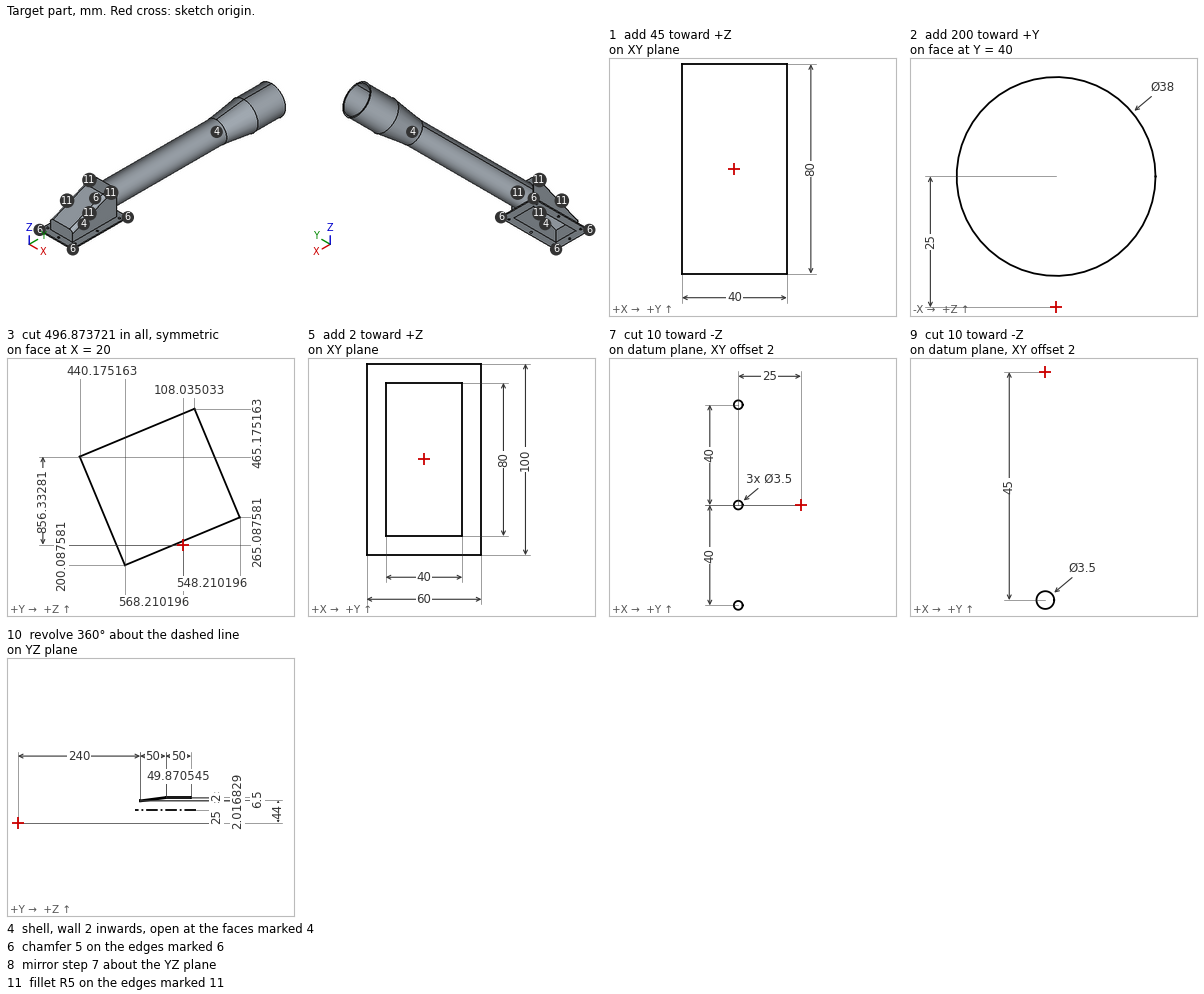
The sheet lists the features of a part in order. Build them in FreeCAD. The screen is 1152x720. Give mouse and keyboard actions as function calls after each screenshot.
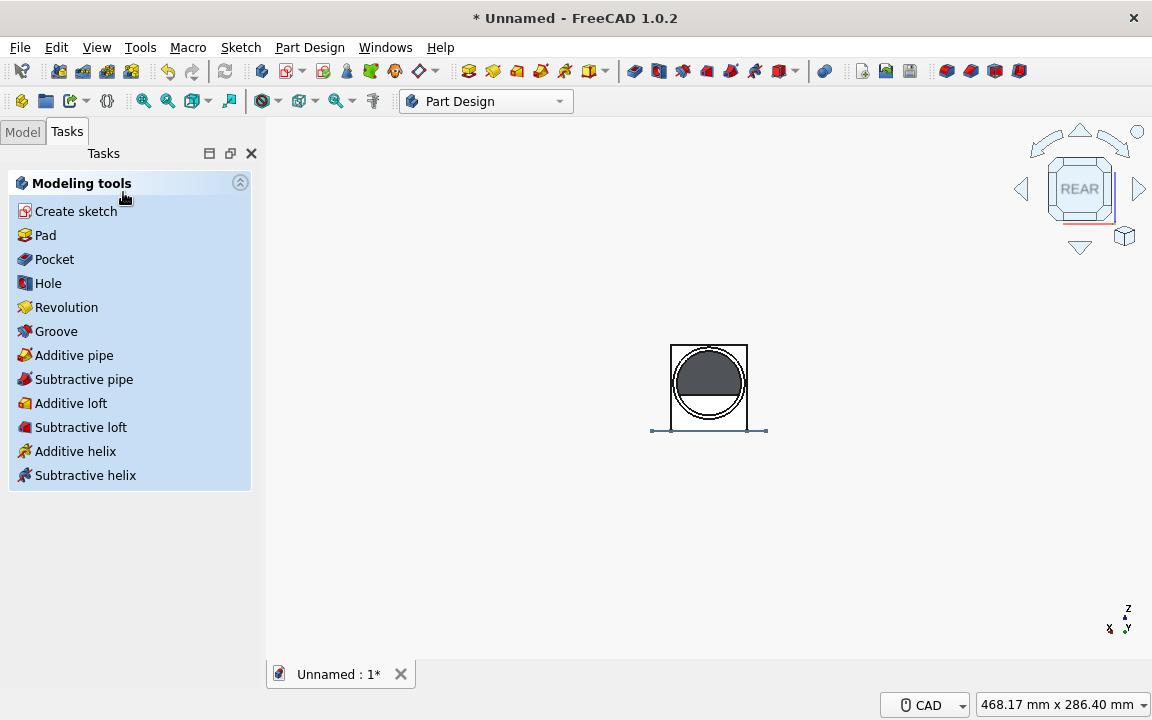
click(470, 72)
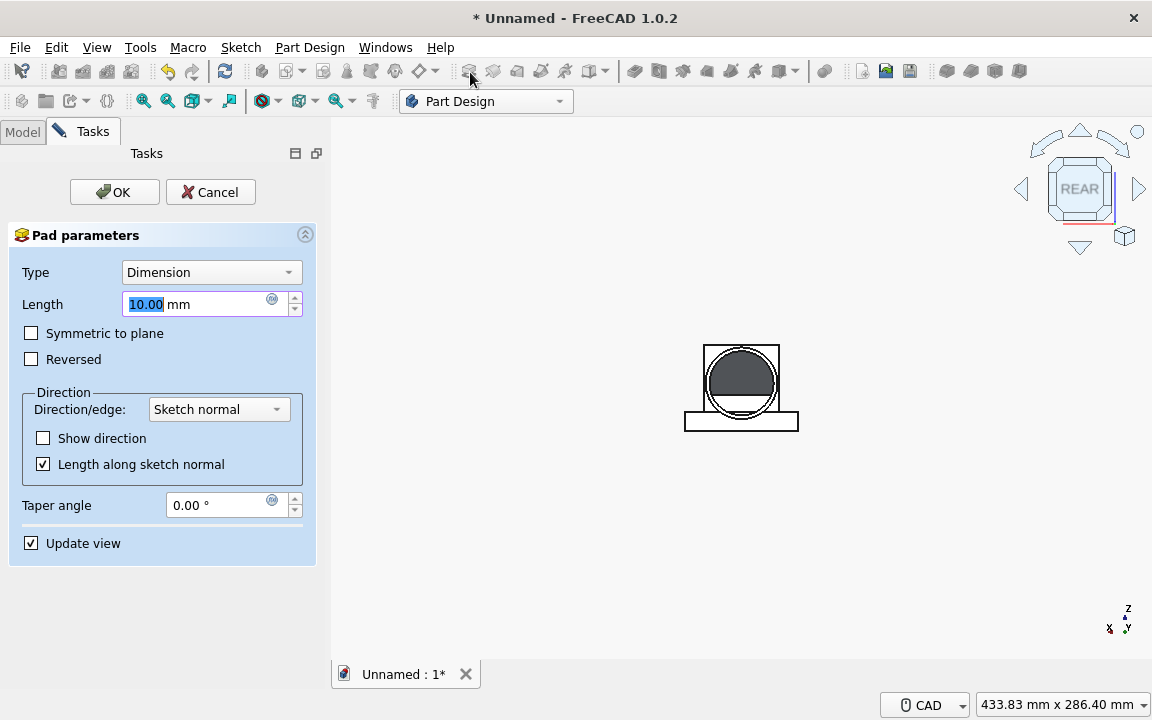
text(2)
key(Tab)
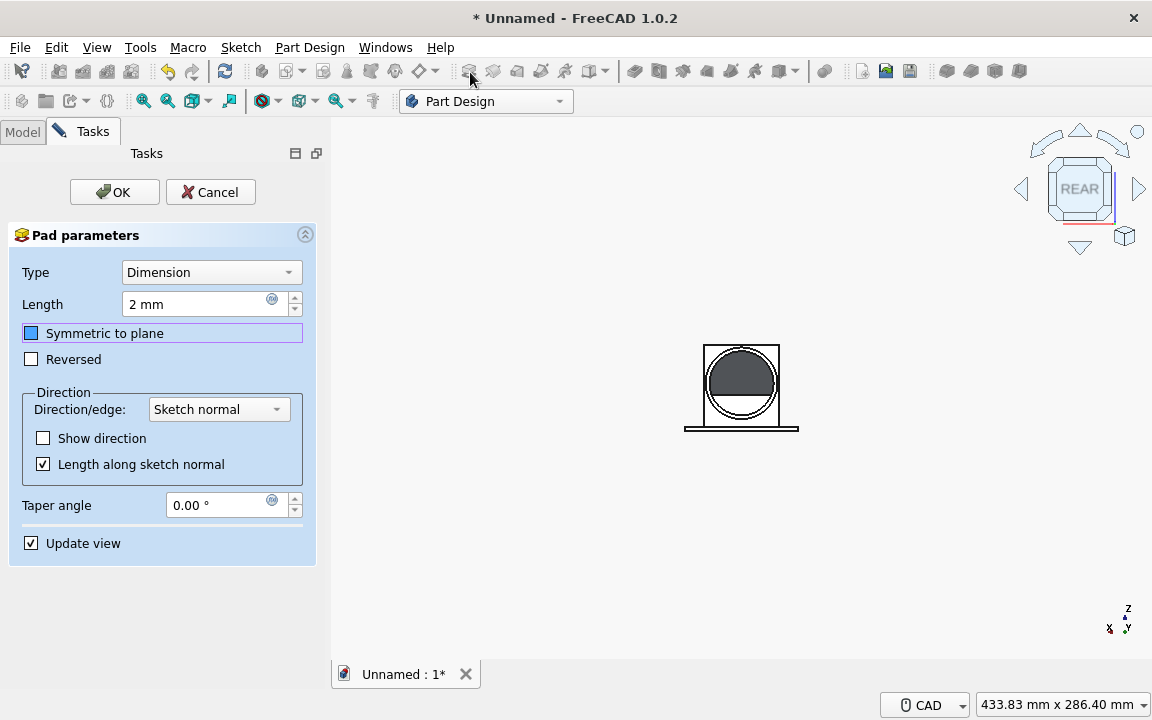
click(115, 192)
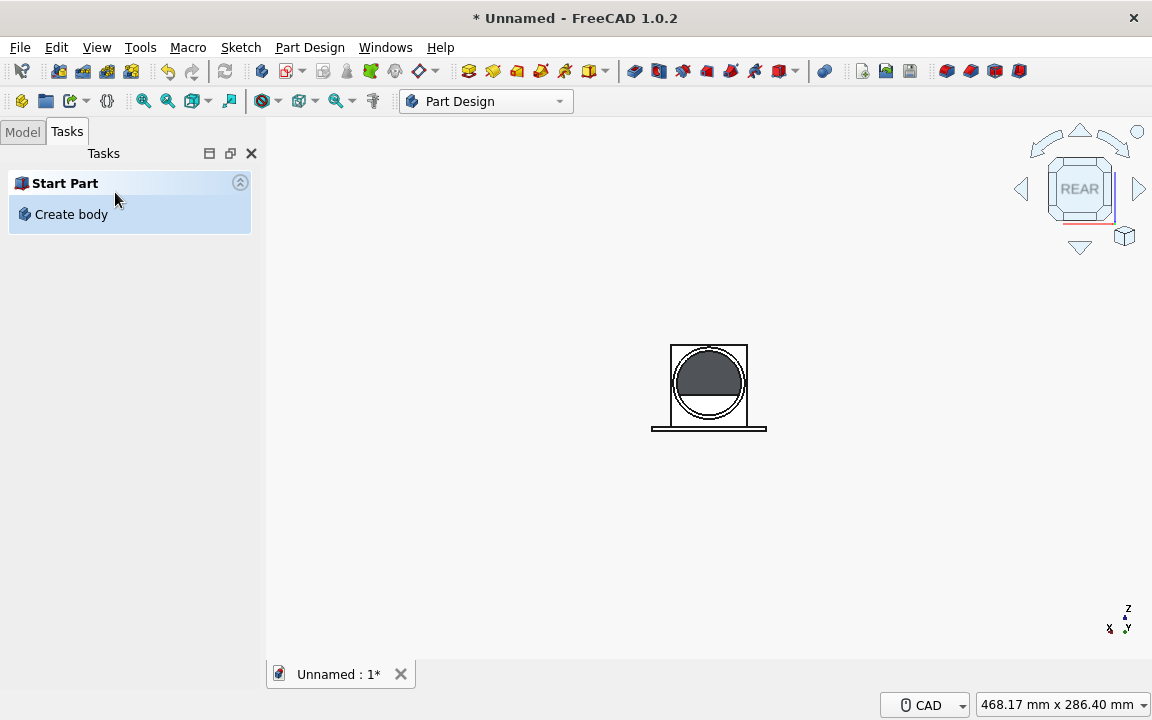
click(144, 102)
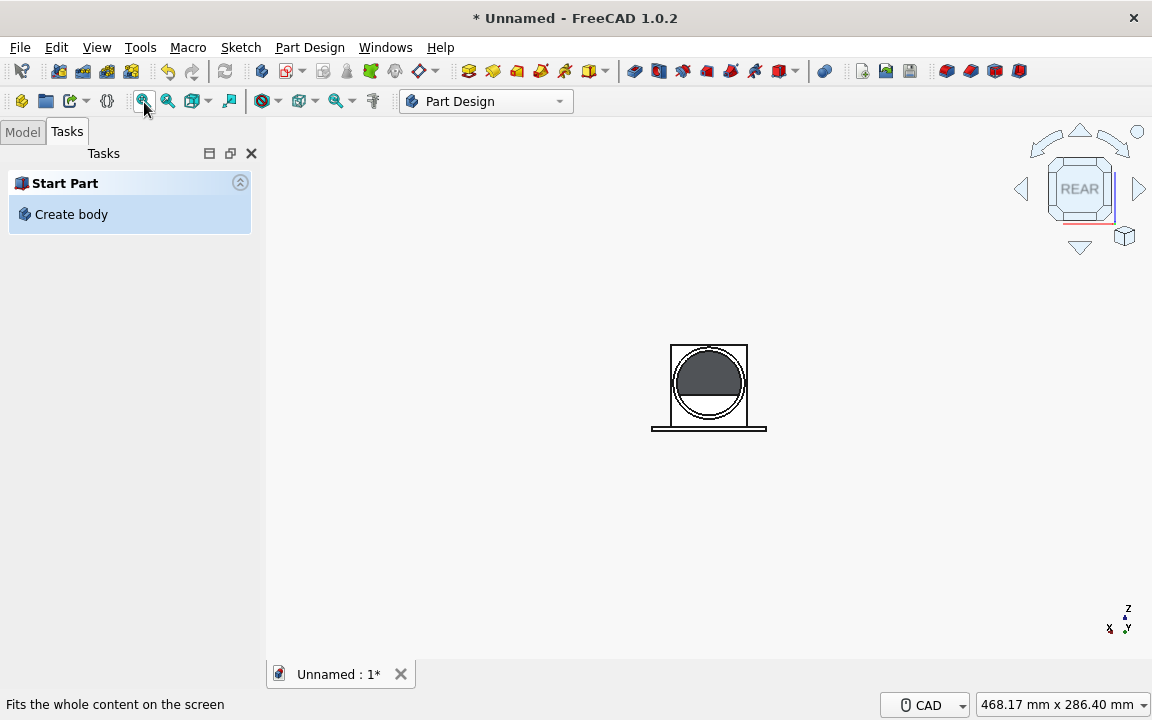
scroll(763, 426, up, 13)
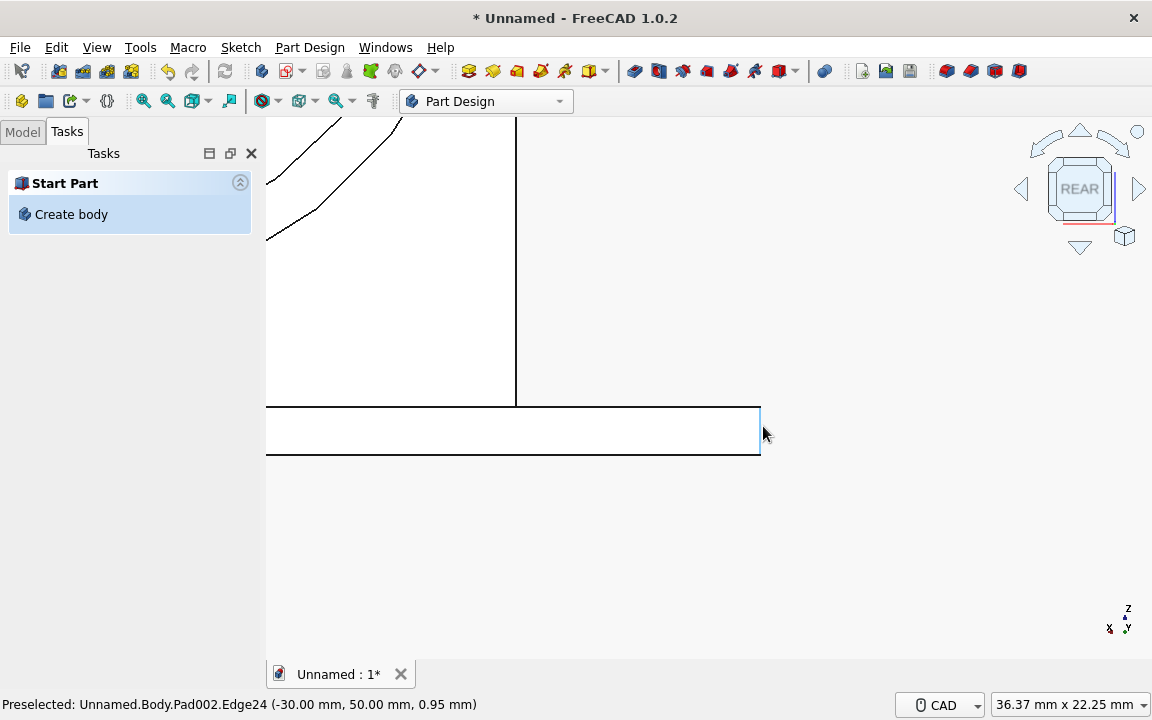
click(760, 430)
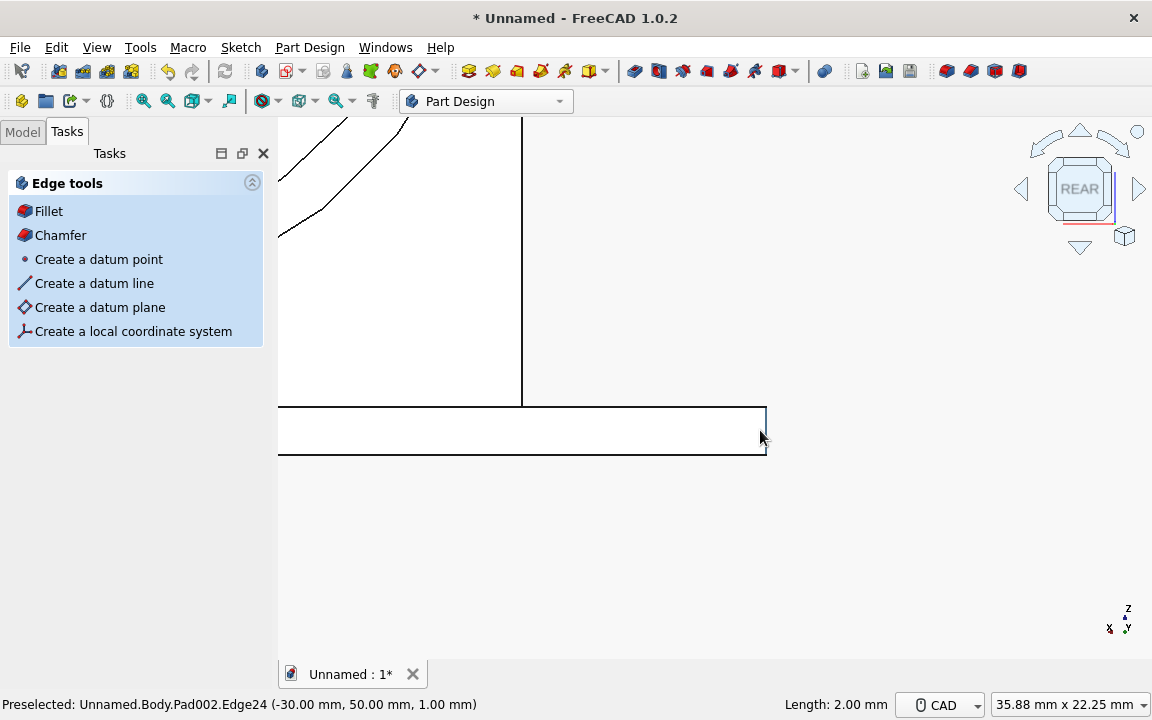
key(v)
key(f)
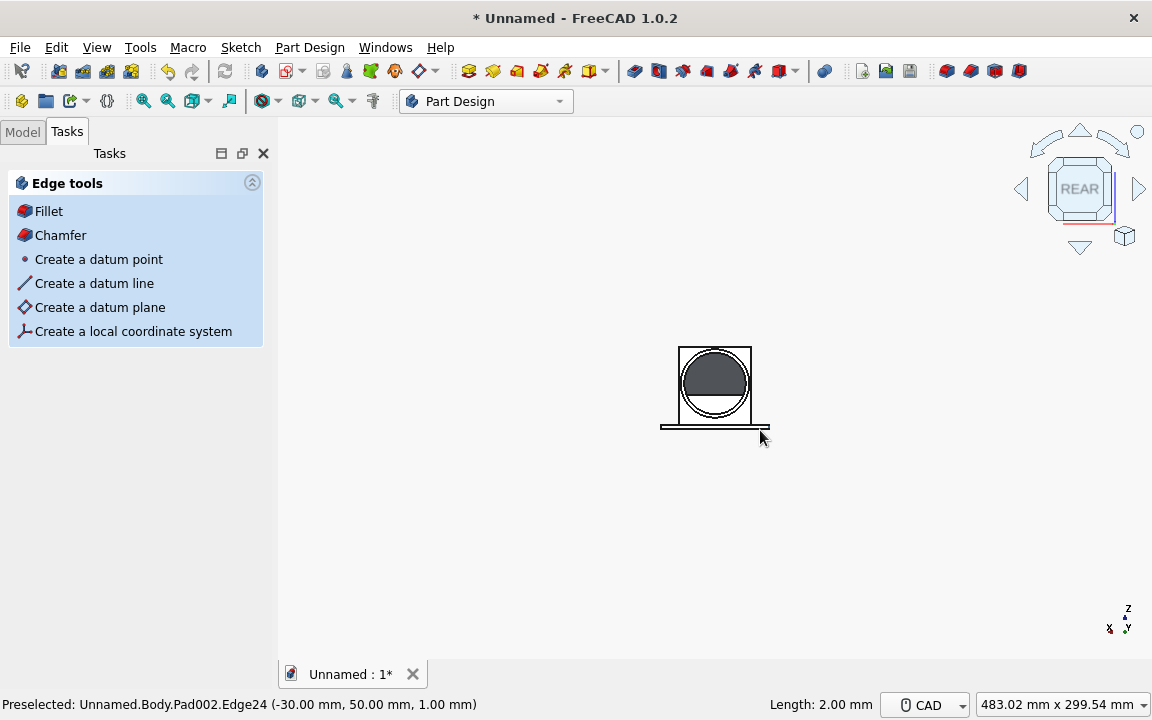
key(0)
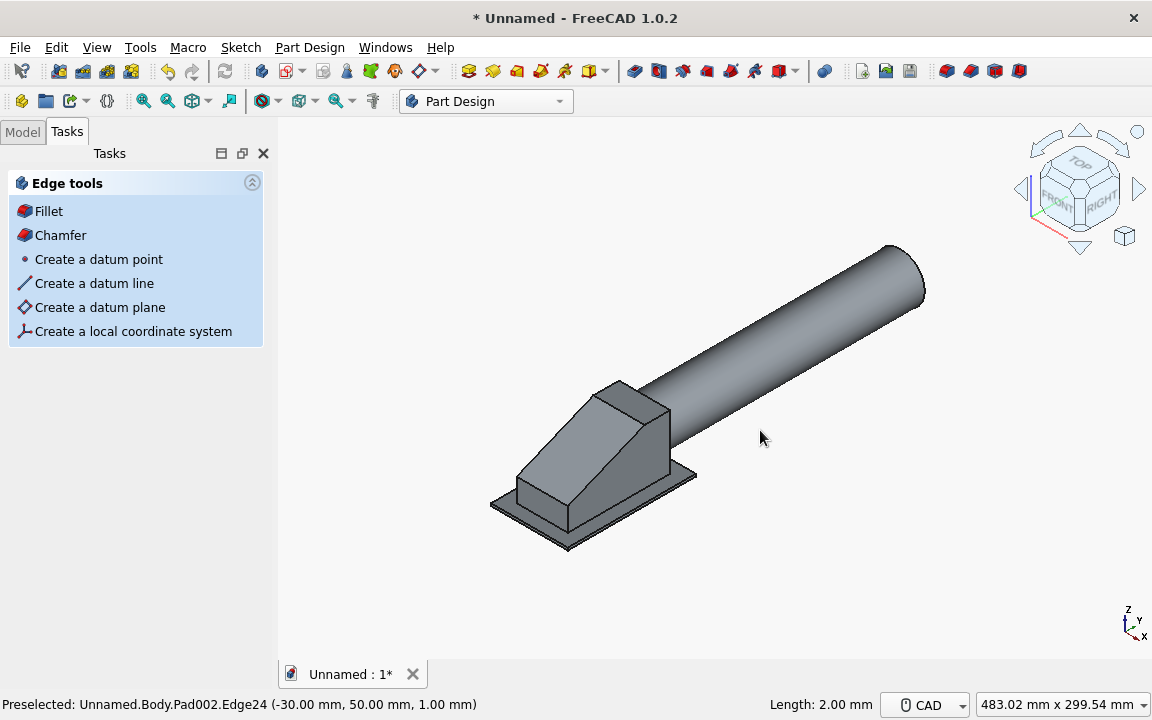
scroll(491, 504, up, 13)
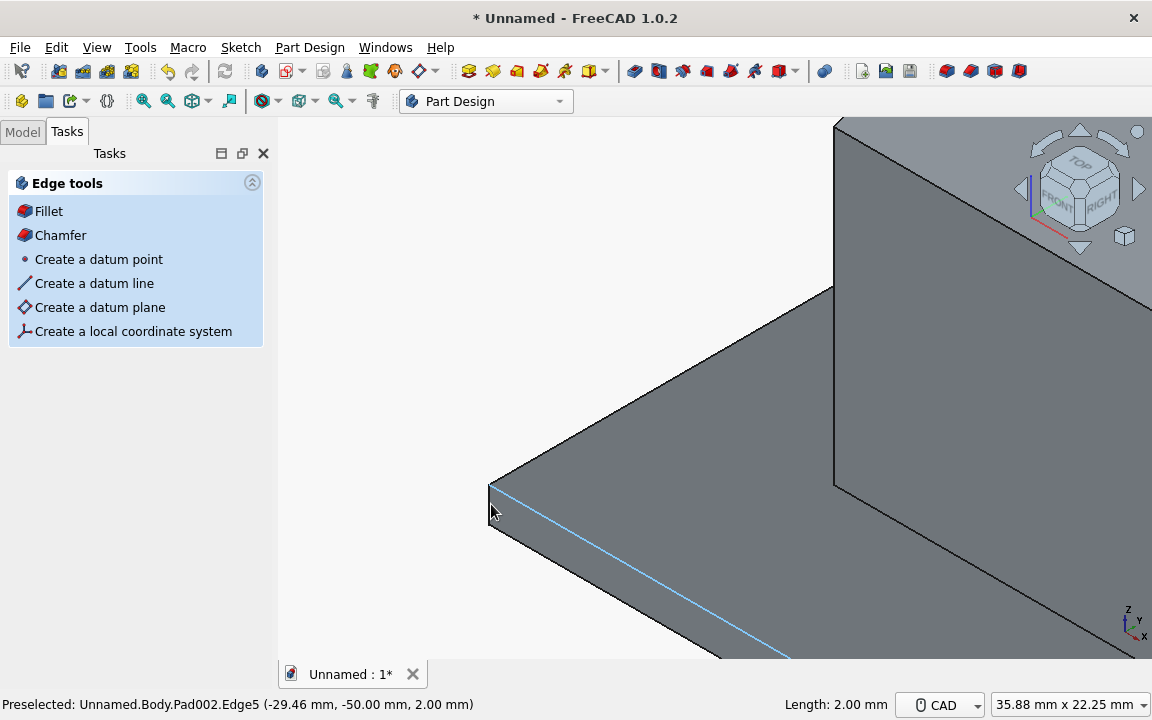
click(144, 102)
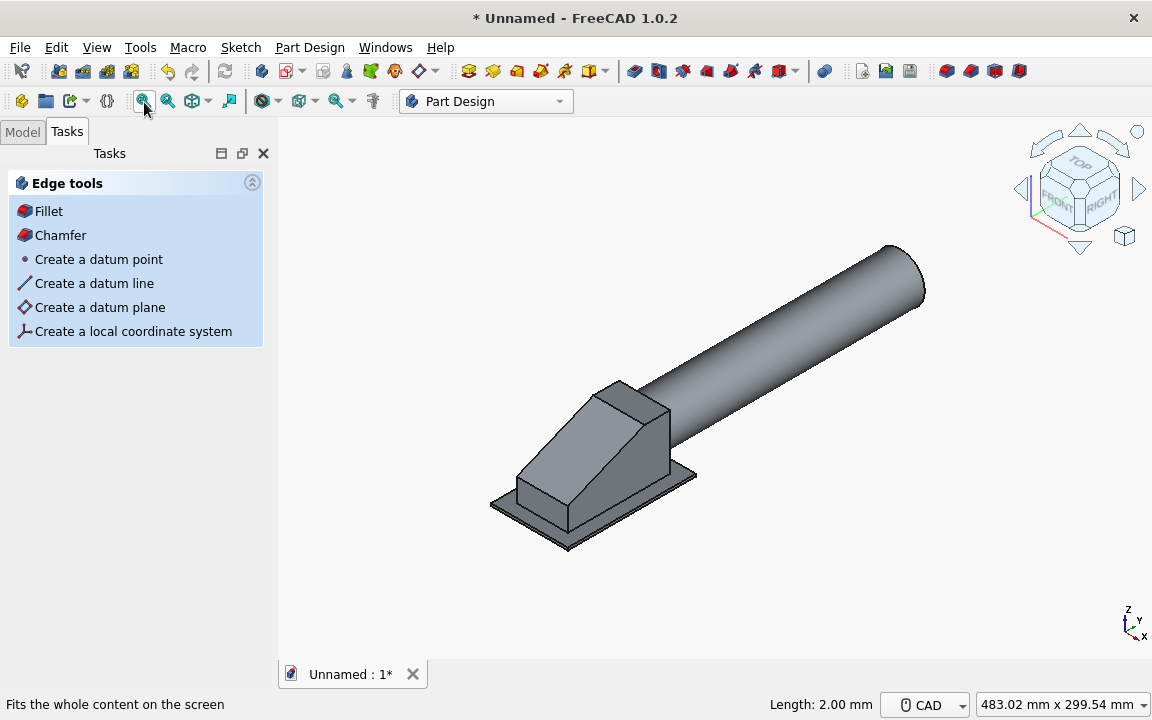
key(2)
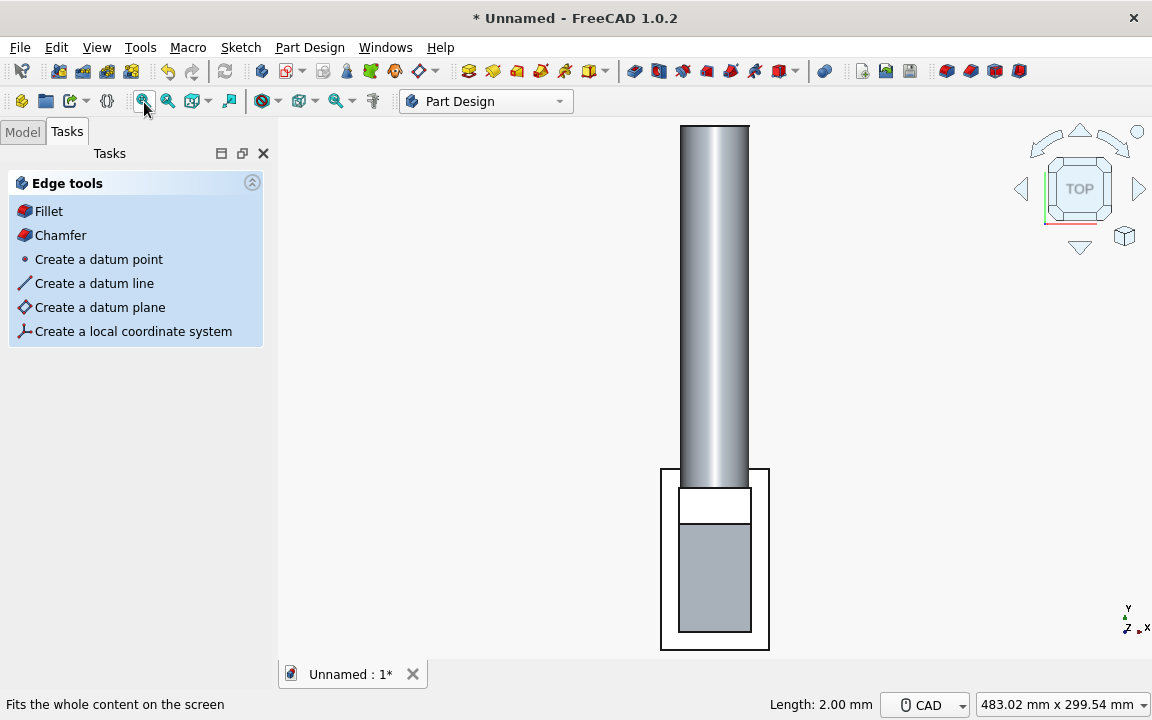
key(1)